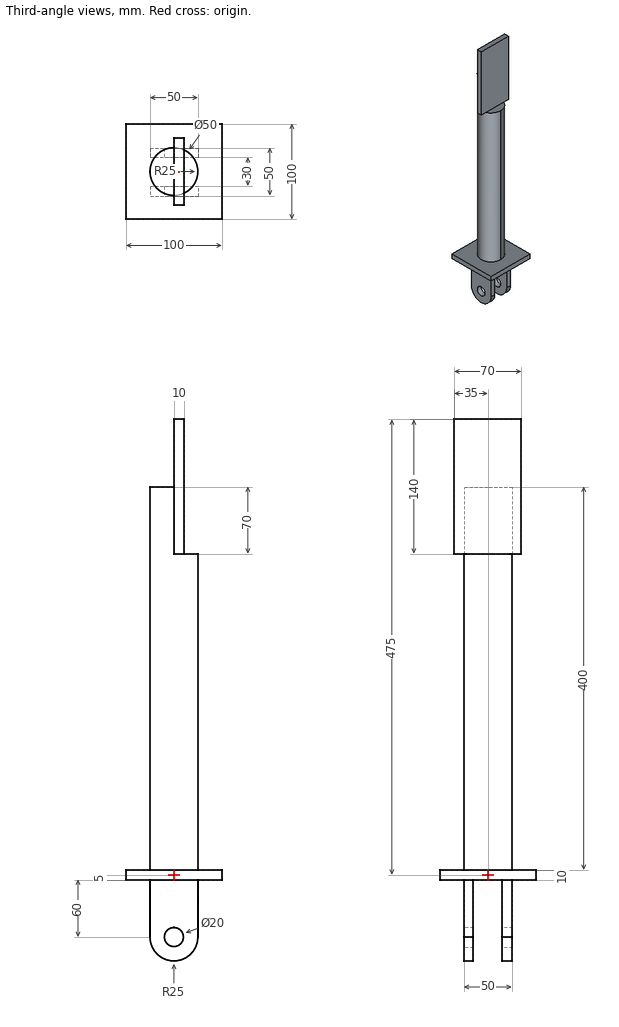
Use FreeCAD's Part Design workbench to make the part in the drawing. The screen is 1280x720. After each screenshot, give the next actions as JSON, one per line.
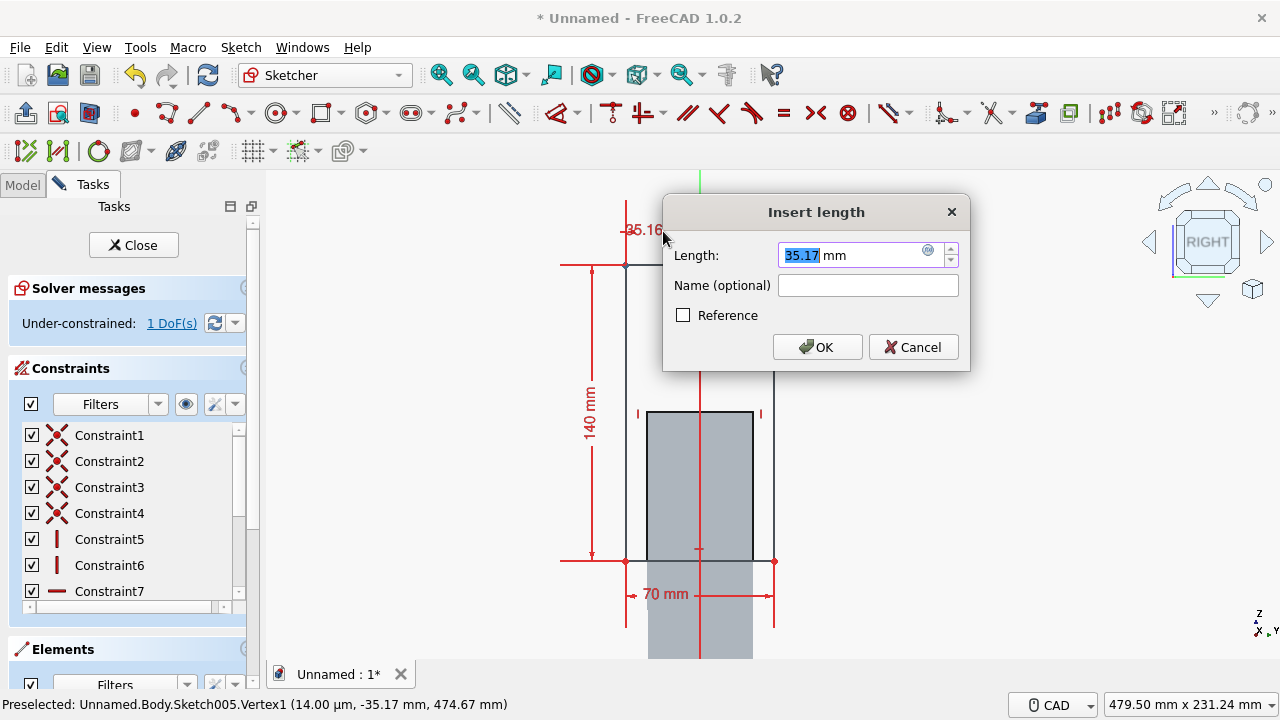
{"action": "type", "text": "35"}
{"action": "key", "text": "Return"}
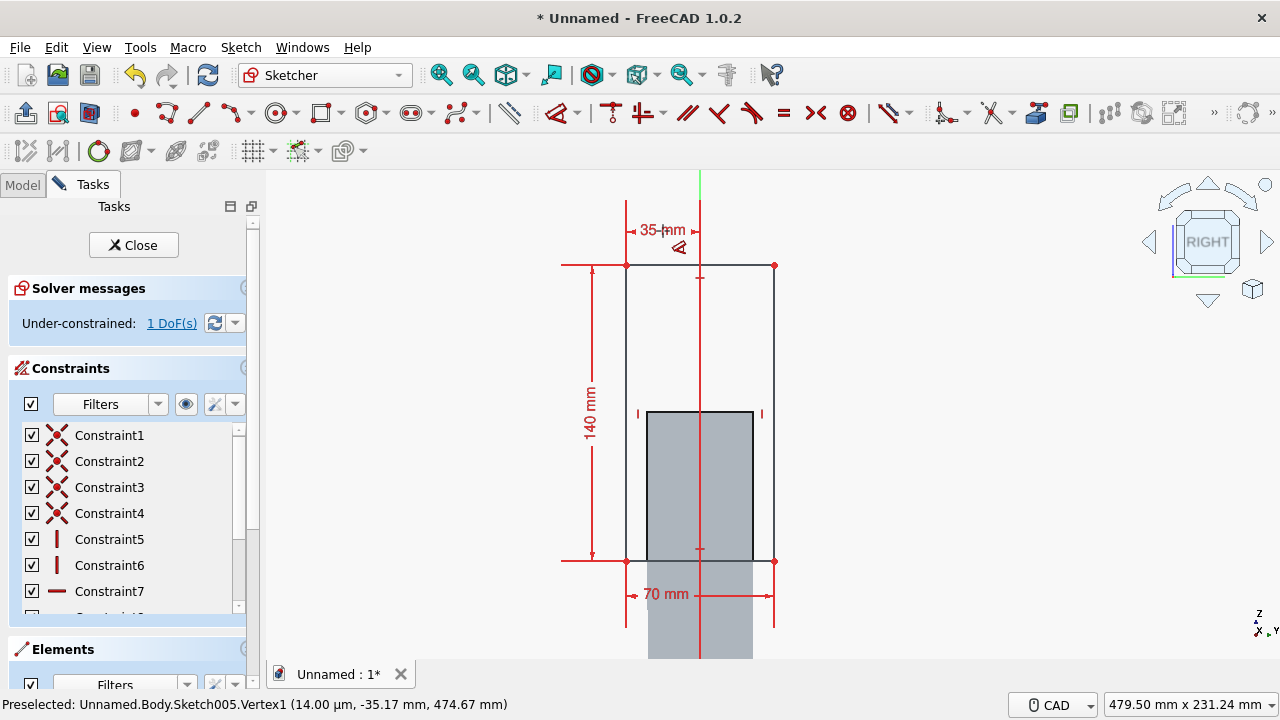
{"action": "left_click", "coordinate": [626, 265]}
{"action": "left_click", "coordinate": [592, 448]}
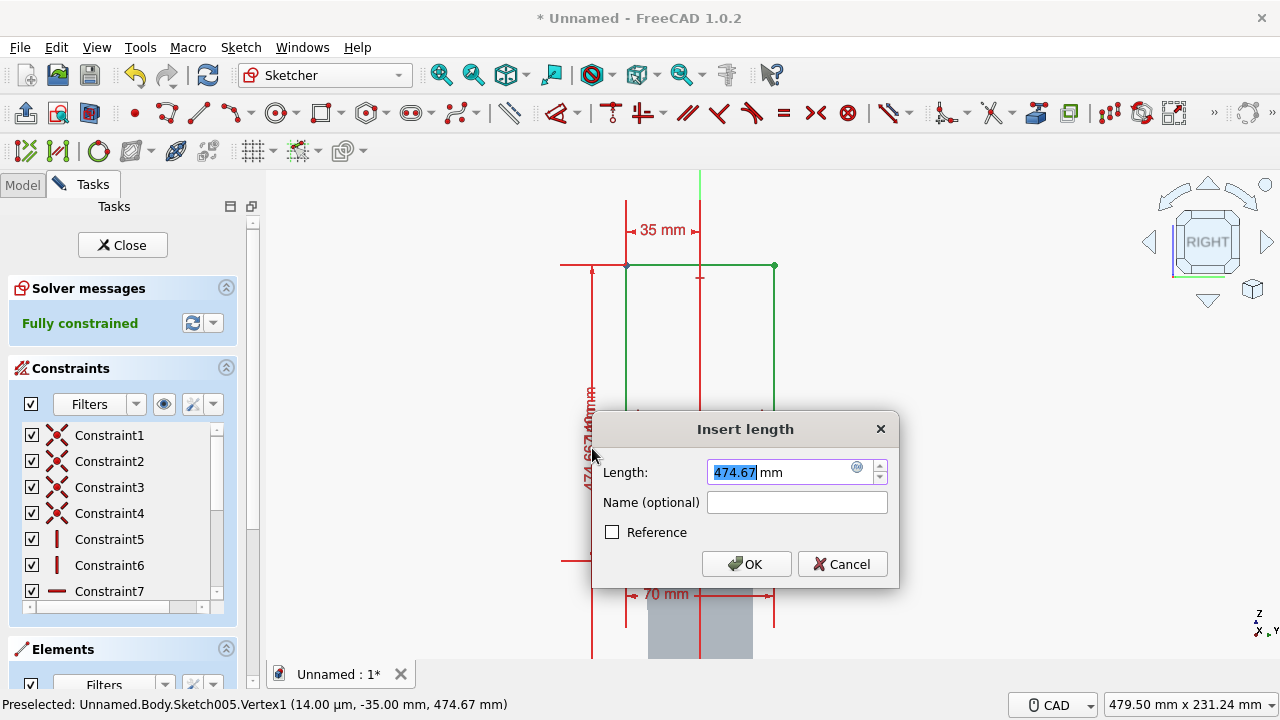
{"action": "type", "text": "475"}
{"action": "key", "text": "Return"}
{"action": "key", "text": "Escape"}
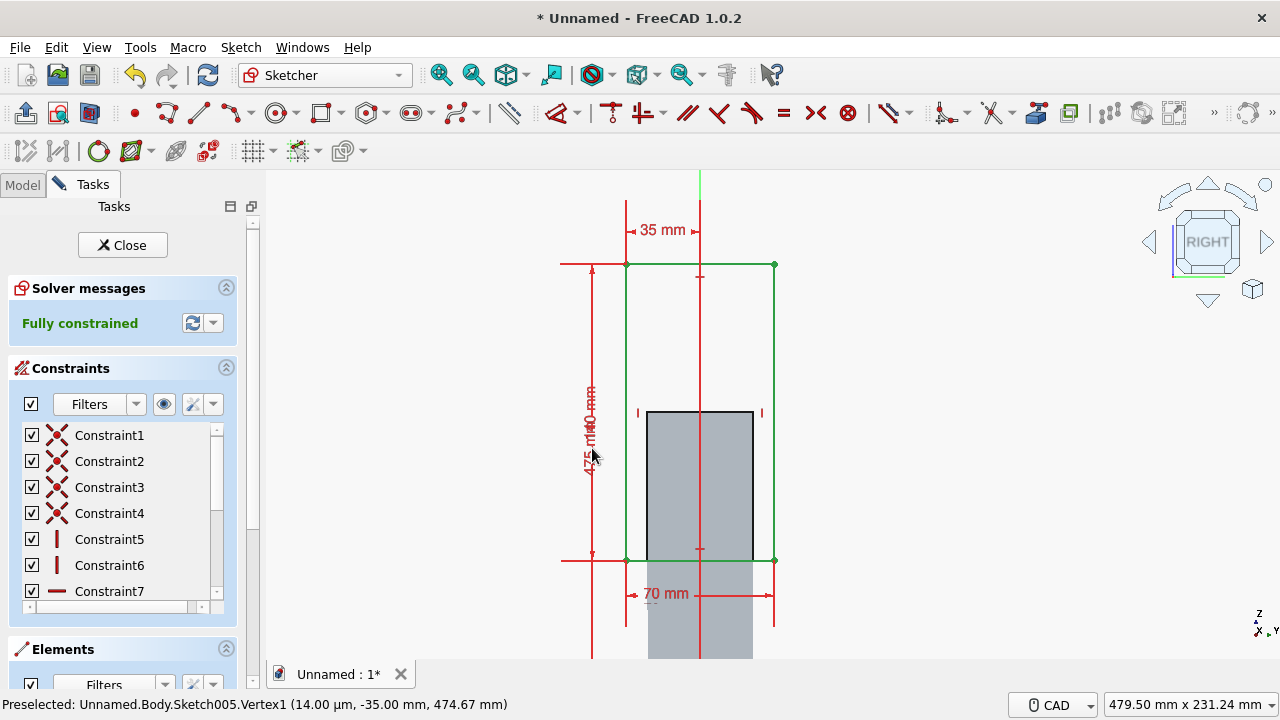
{"action": "left_click", "coordinate": [123, 245]}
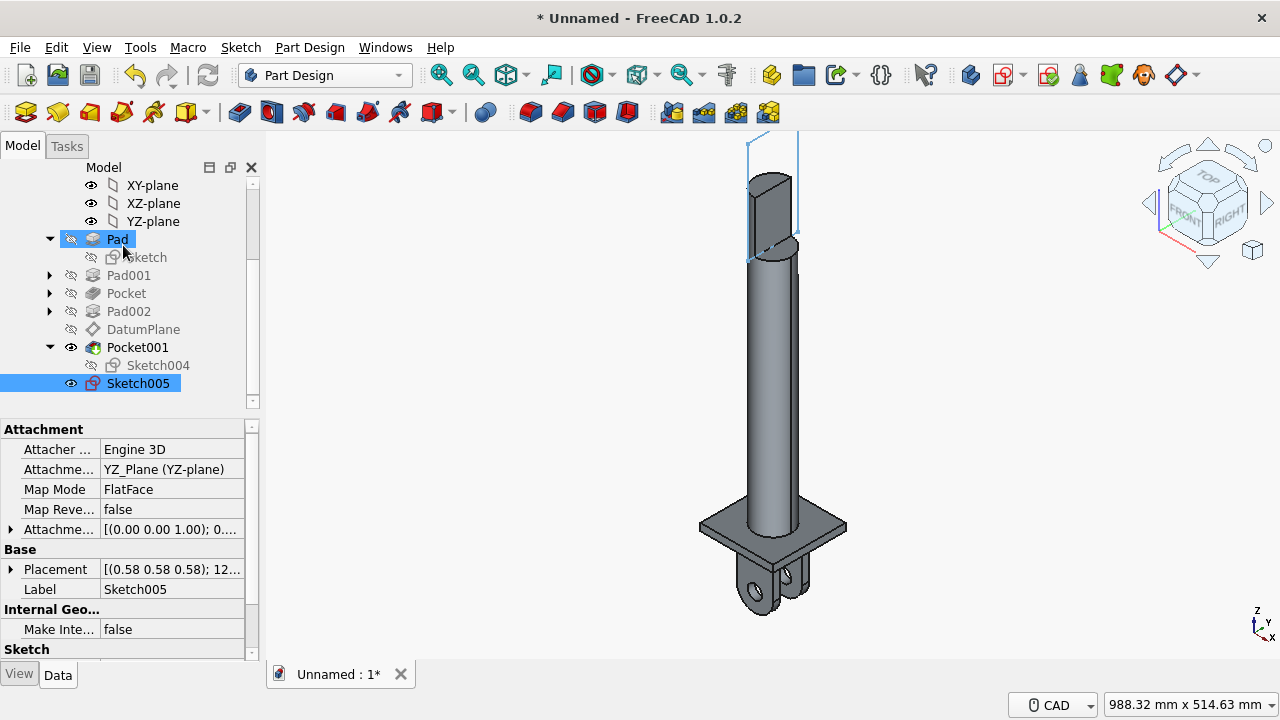
{"action": "left_click", "coordinate": [26, 112]}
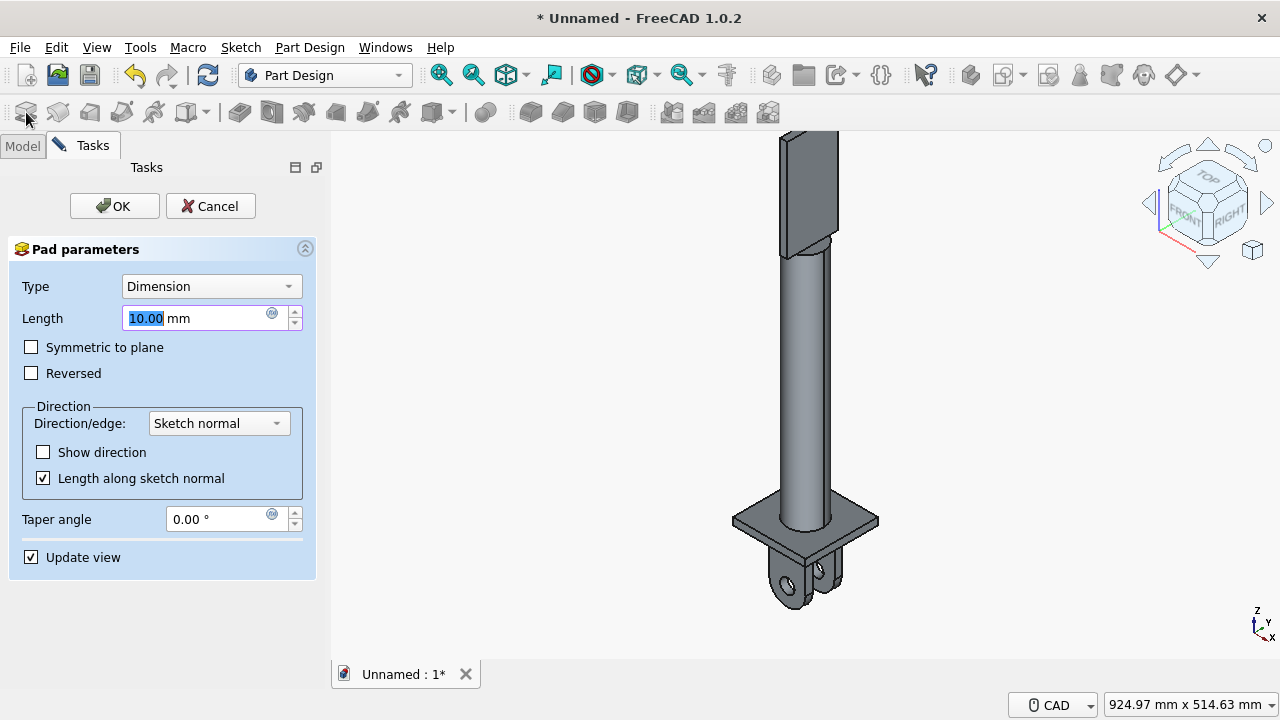
{"action": "type", "text": "10"}
{"action": "key", "text": "Tab"}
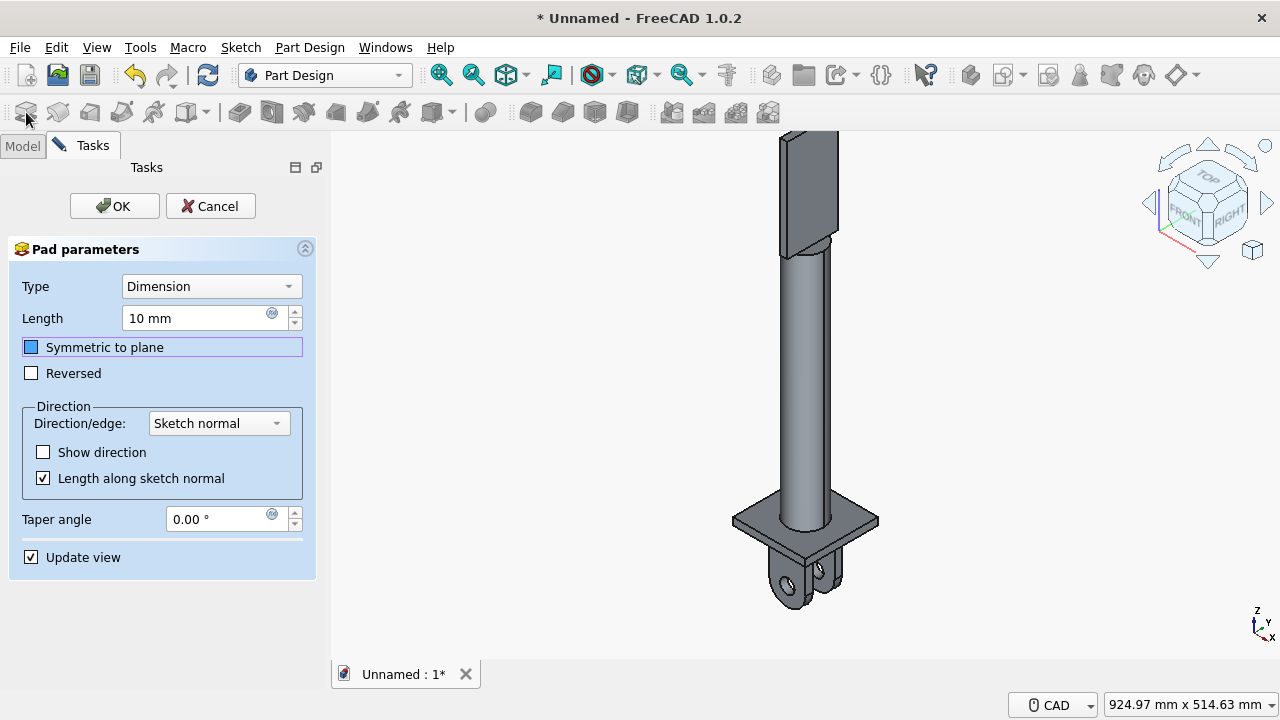
{"action": "left_click", "coordinate": [115, 206]}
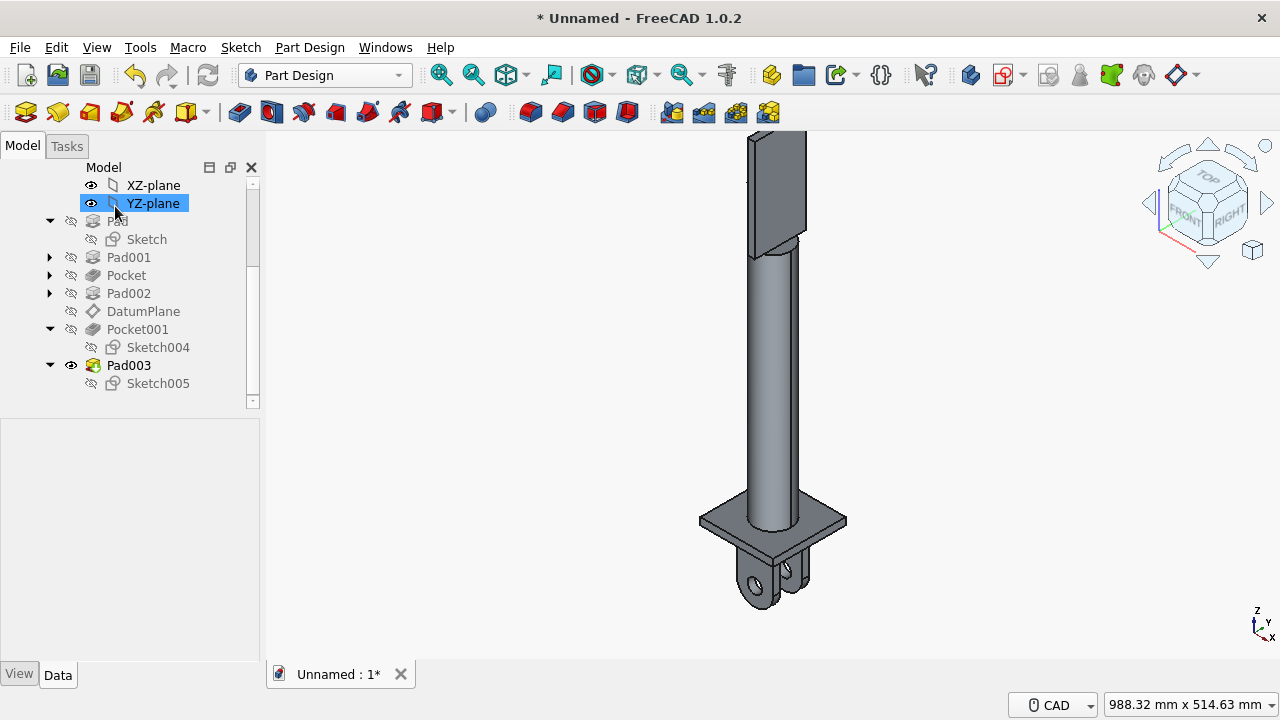
{"action": "key", "text": "v f"}